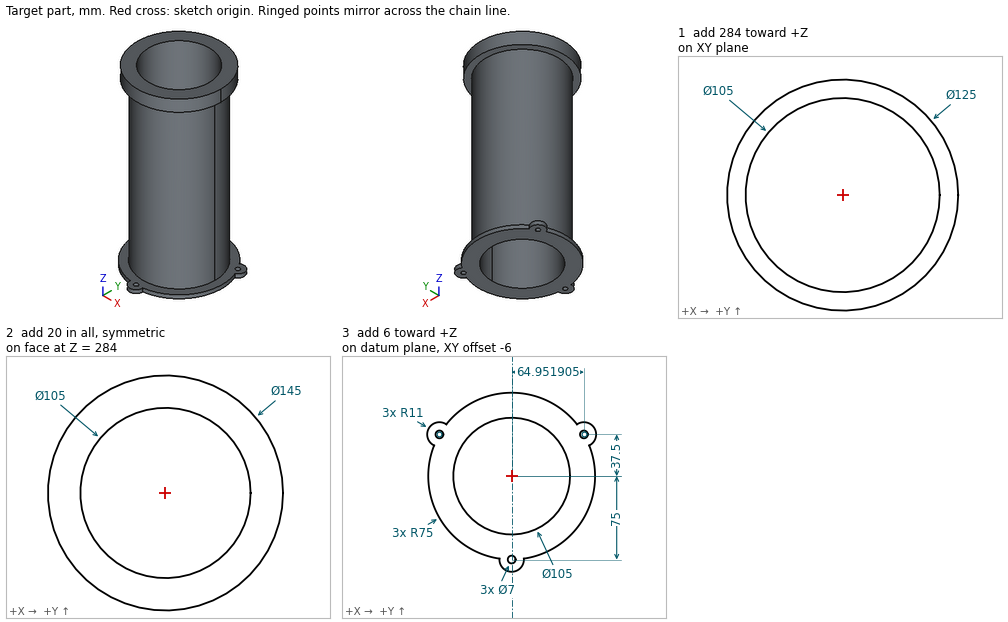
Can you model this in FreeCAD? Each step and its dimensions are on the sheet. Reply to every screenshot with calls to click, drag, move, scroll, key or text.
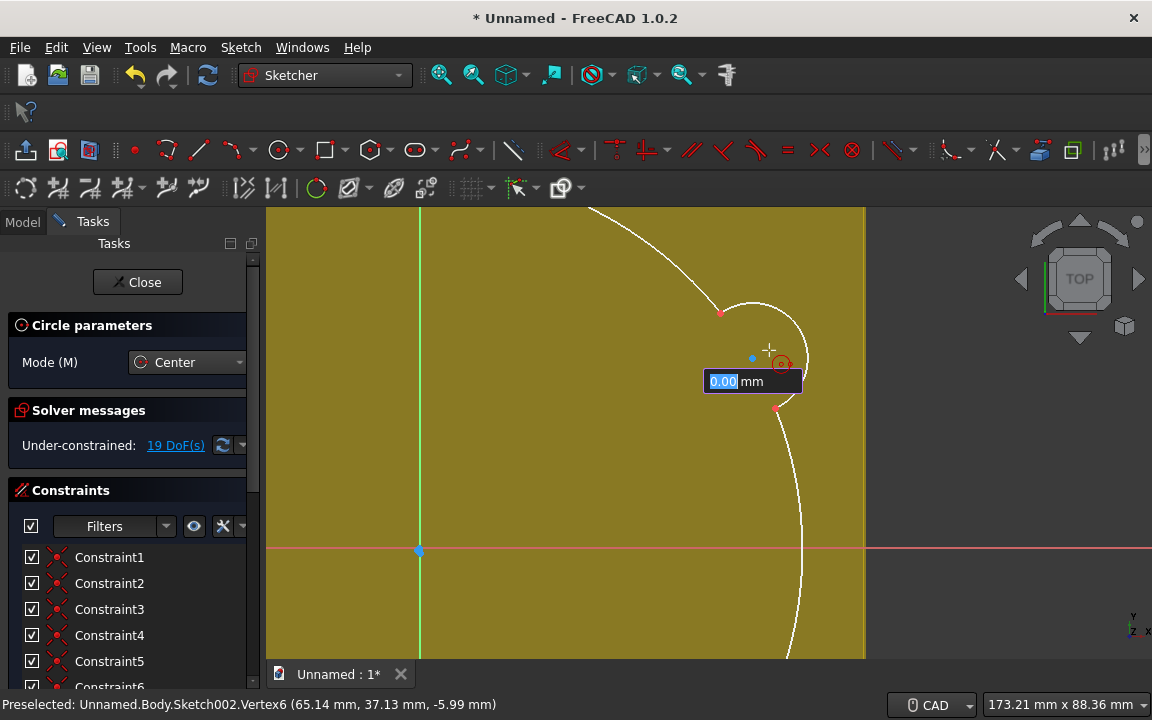
click(769, 350)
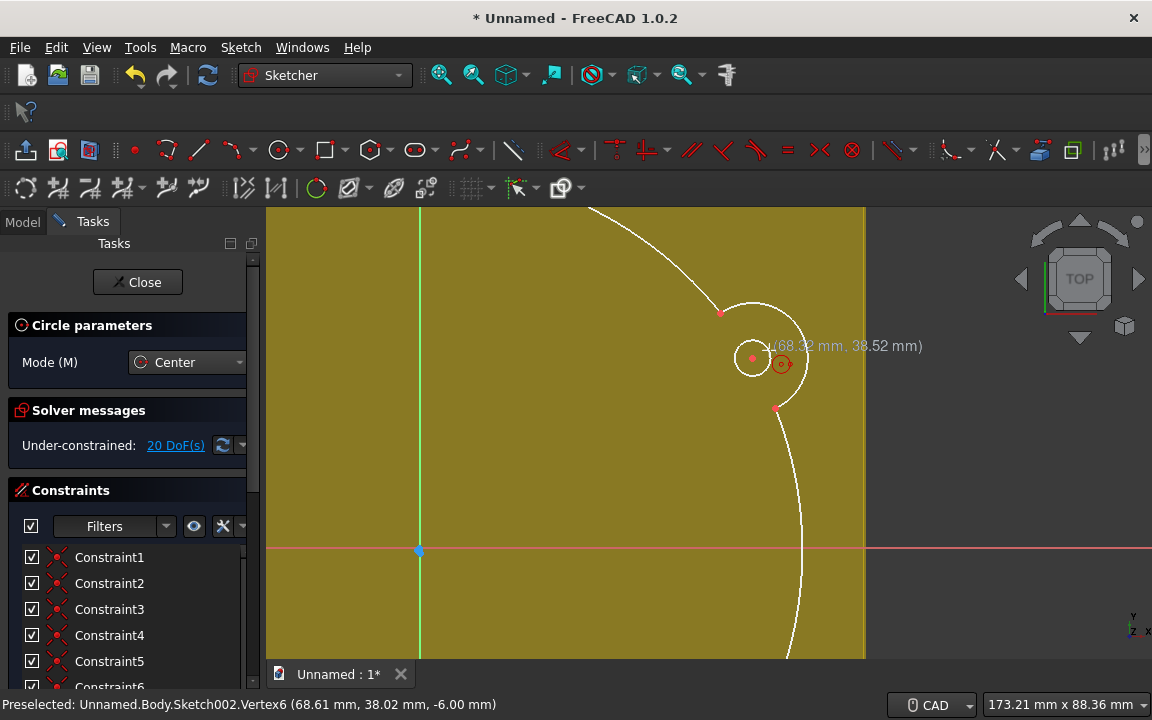
click(420, 548)
click(609, 358)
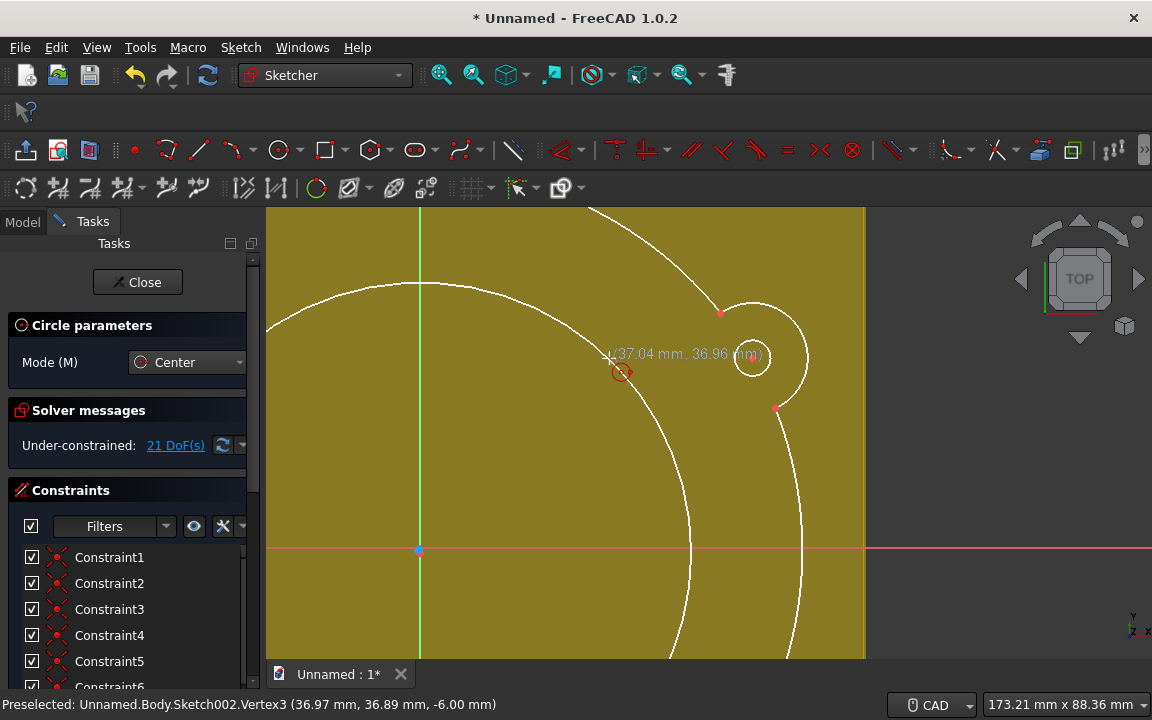
scroll(769, 350, down, 5)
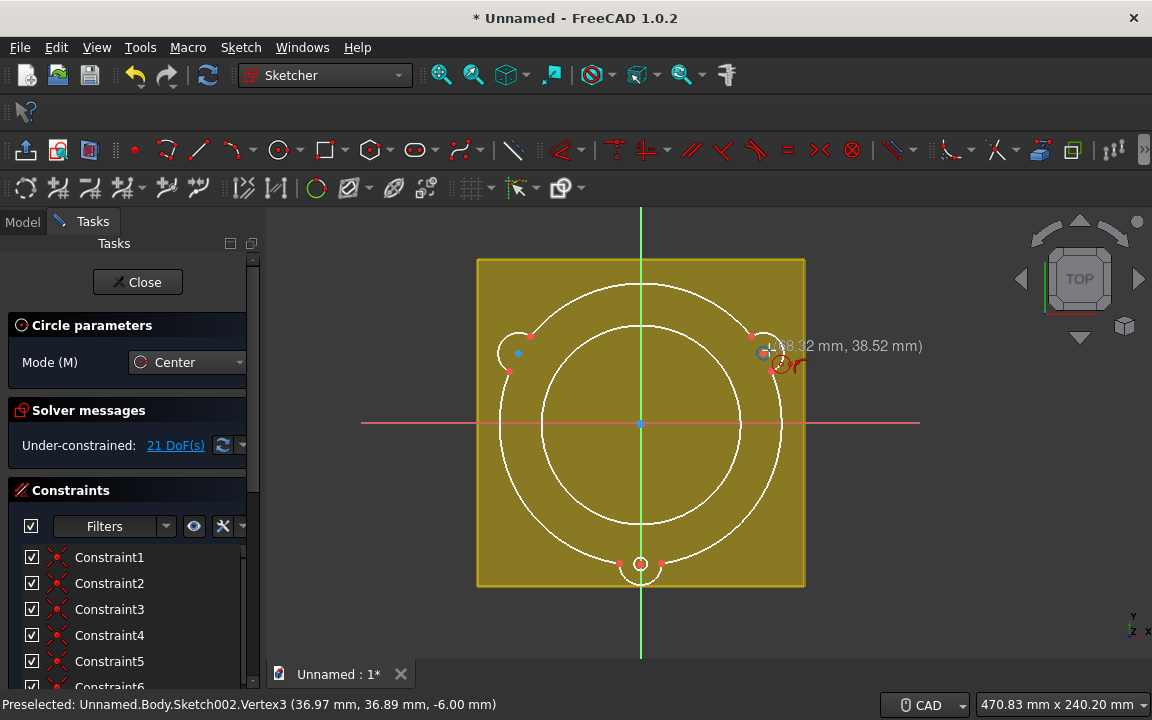
scroll(519, 352, up, 7)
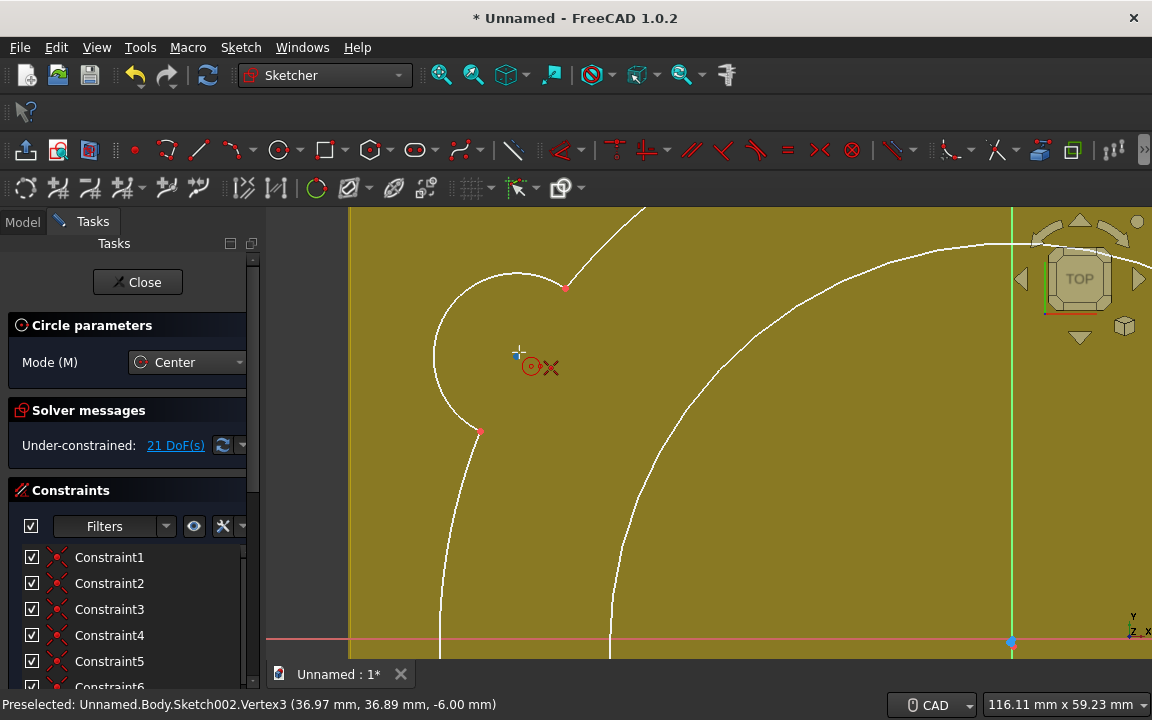
scroll(519, 352, down, 7)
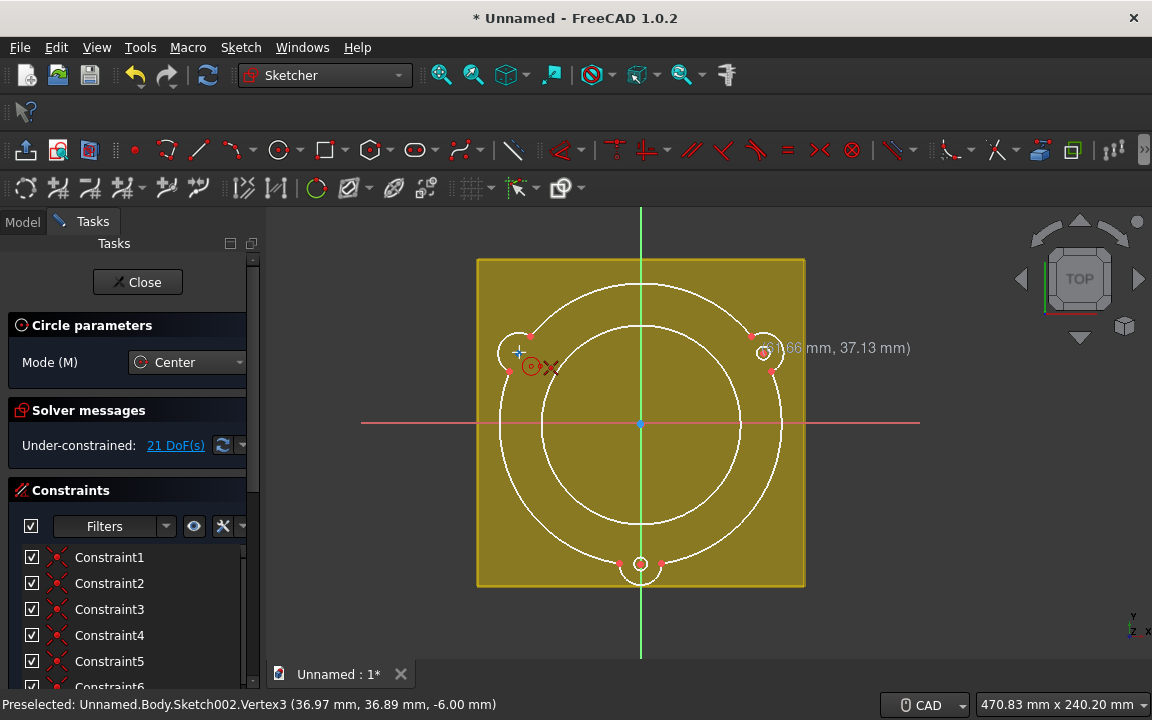
click(519, 352)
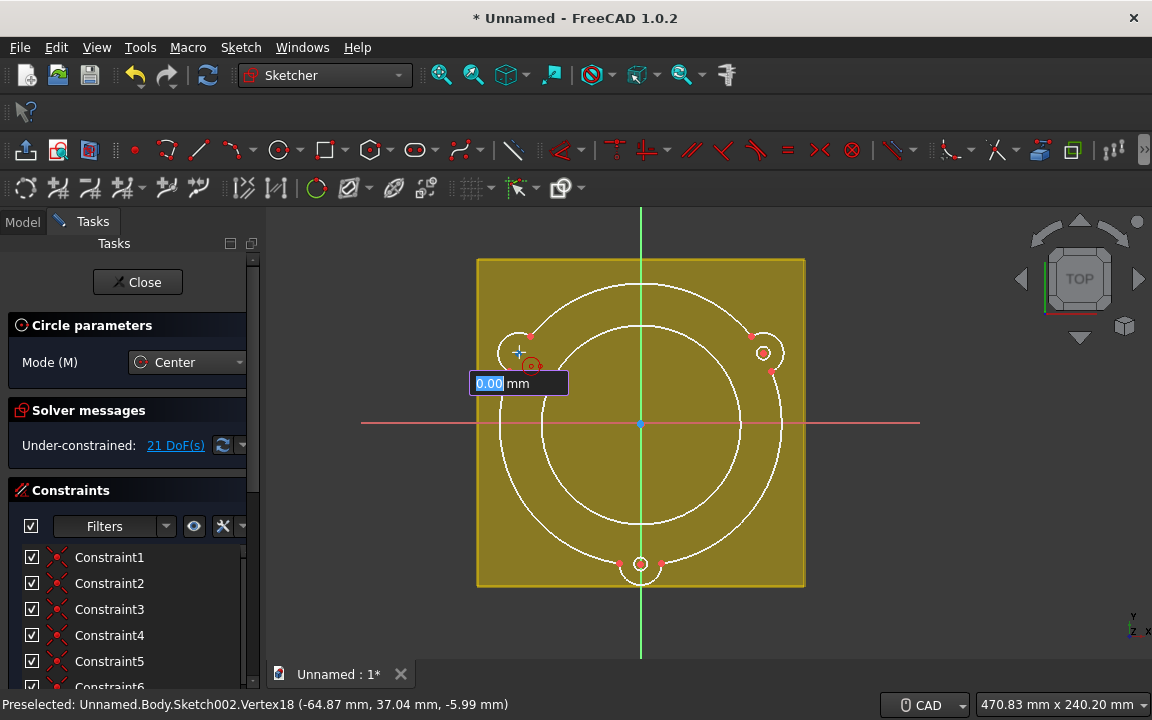
scroll(525, 350, up, 5)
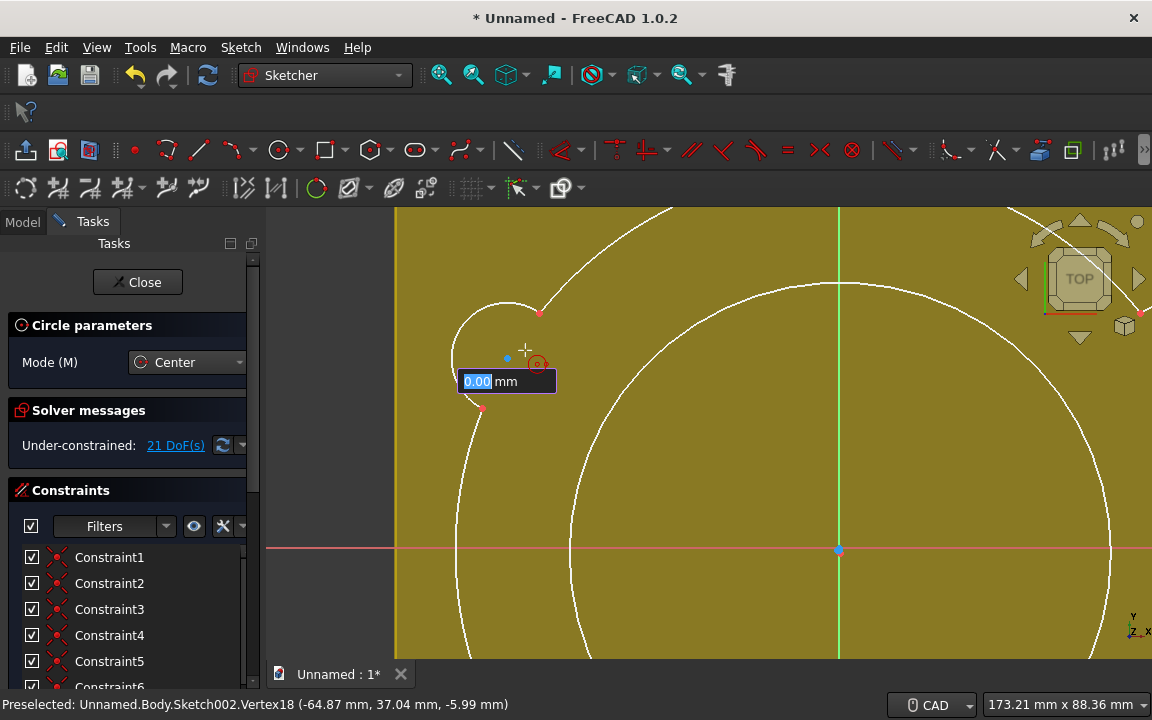
click(524, 350)
key(Escape)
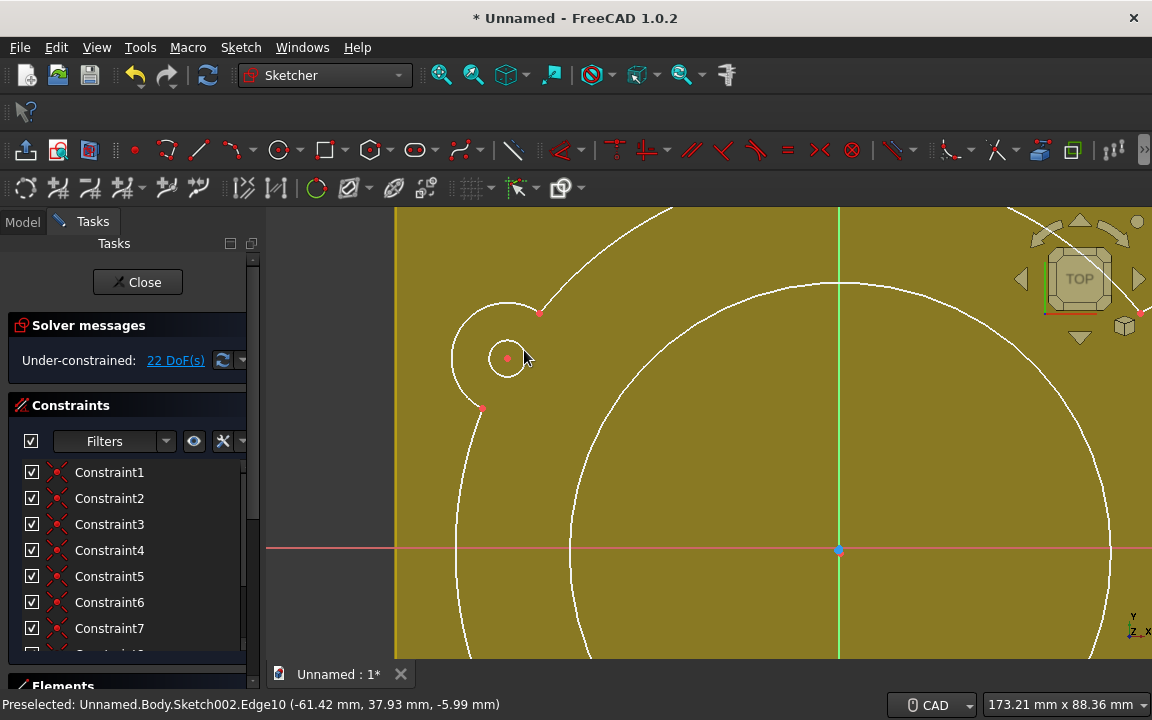
click(648, 362)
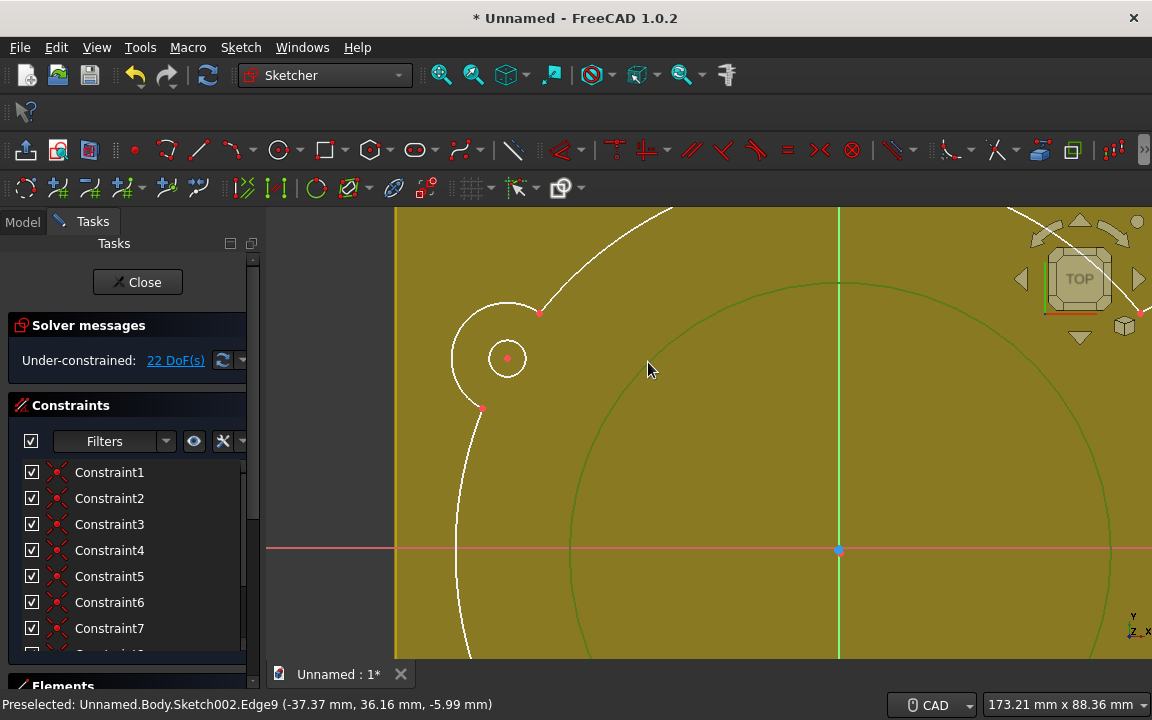
scroll(525, 350, down, 5)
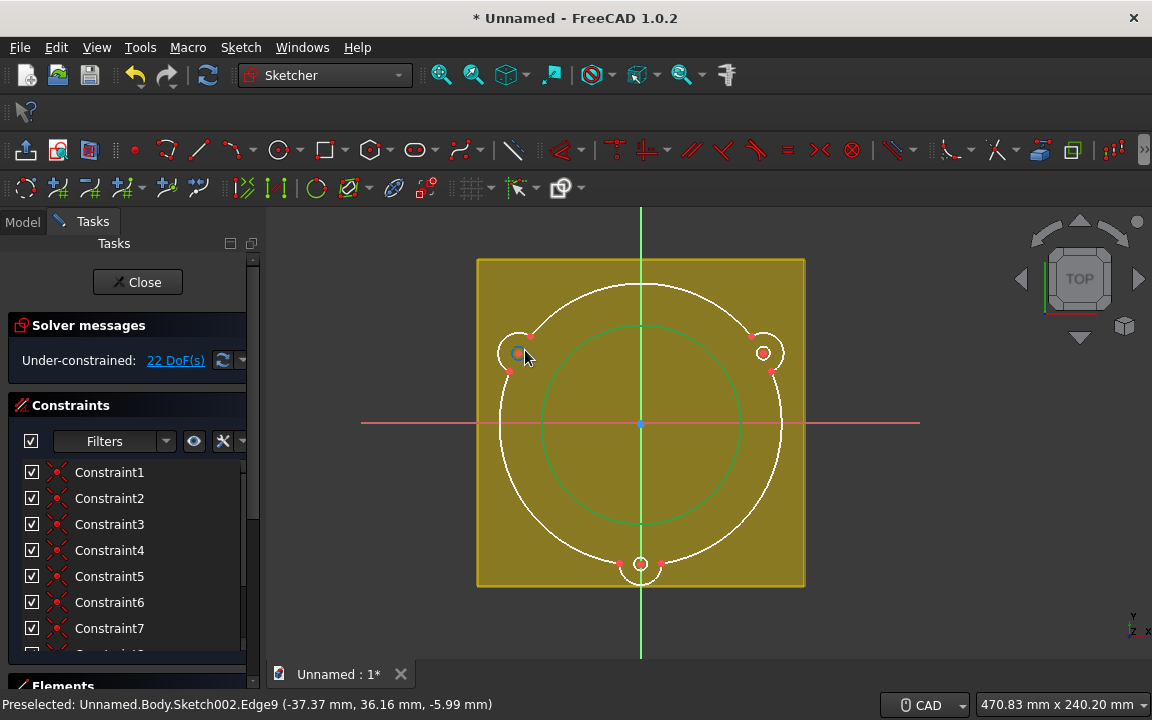
click(730, 533)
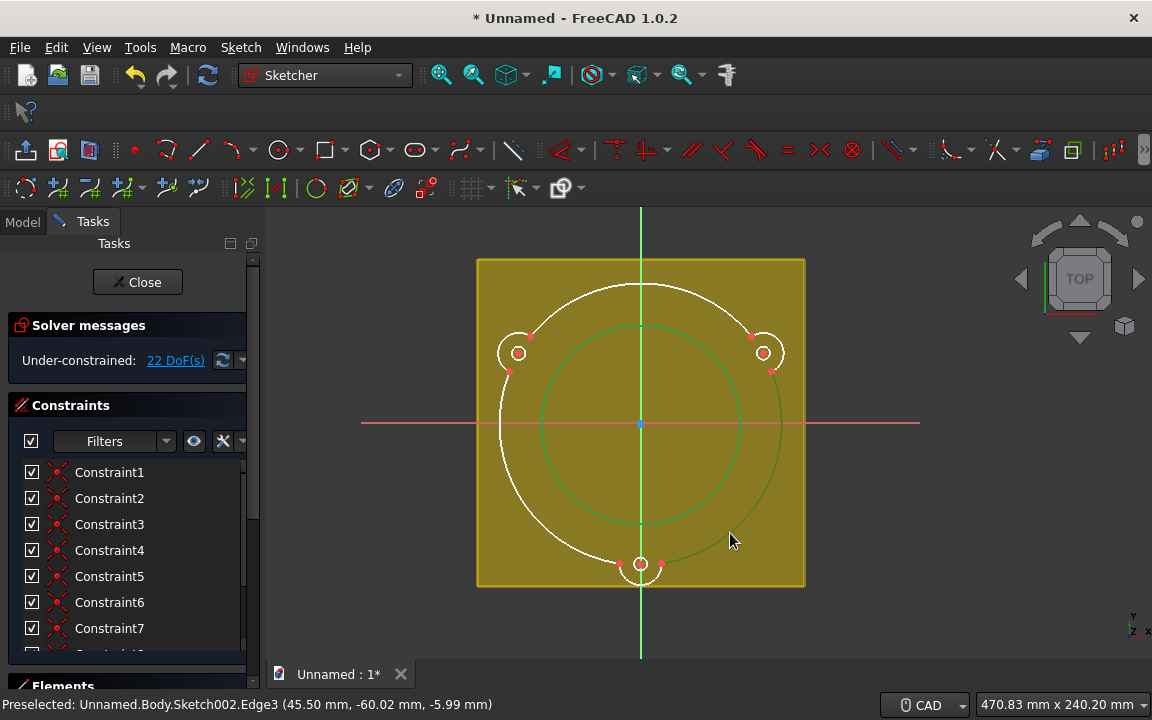
click(616, 150)